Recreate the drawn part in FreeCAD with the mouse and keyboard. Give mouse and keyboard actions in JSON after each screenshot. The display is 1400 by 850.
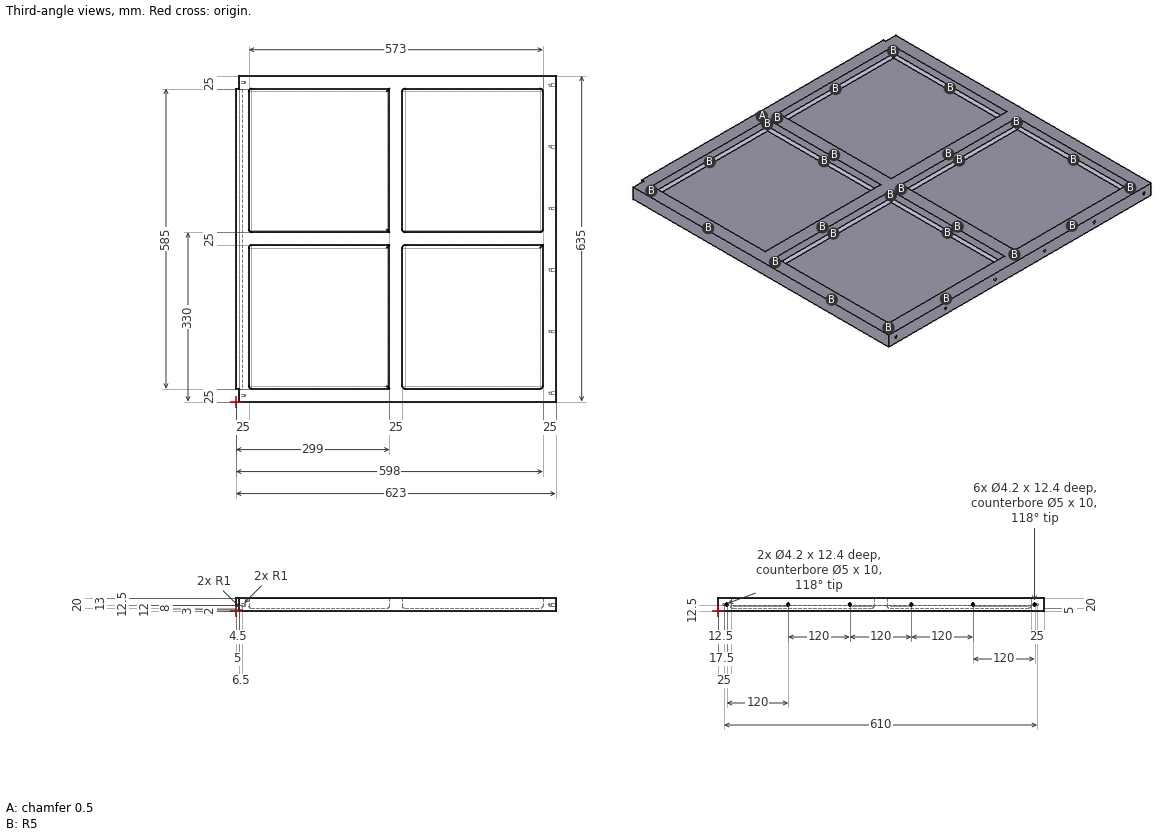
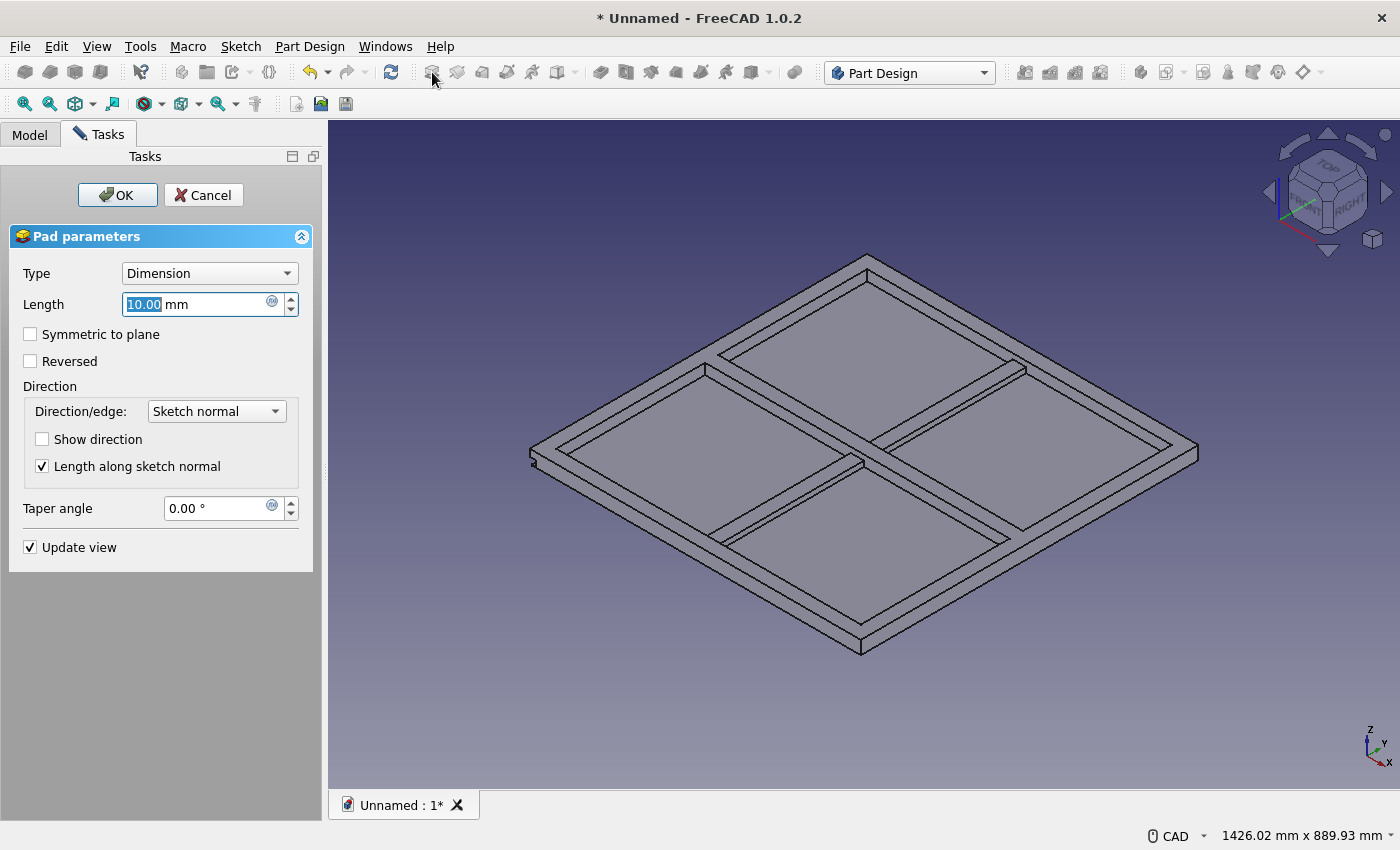
{"action": "type", "text": "20"}
{"action": "key", "text": "Tab"}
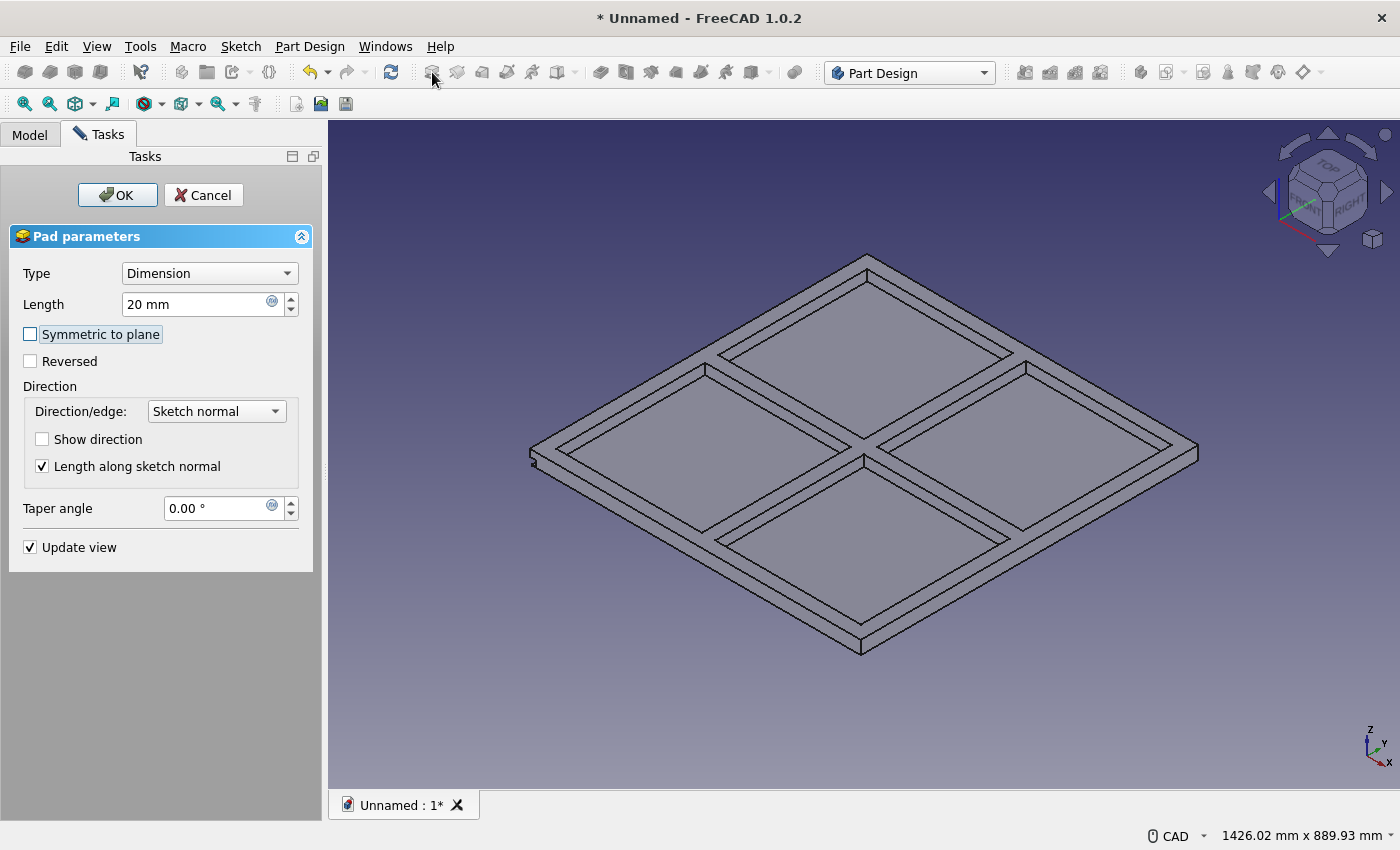
{"action": "left_click", "coordinate": [118, 195]}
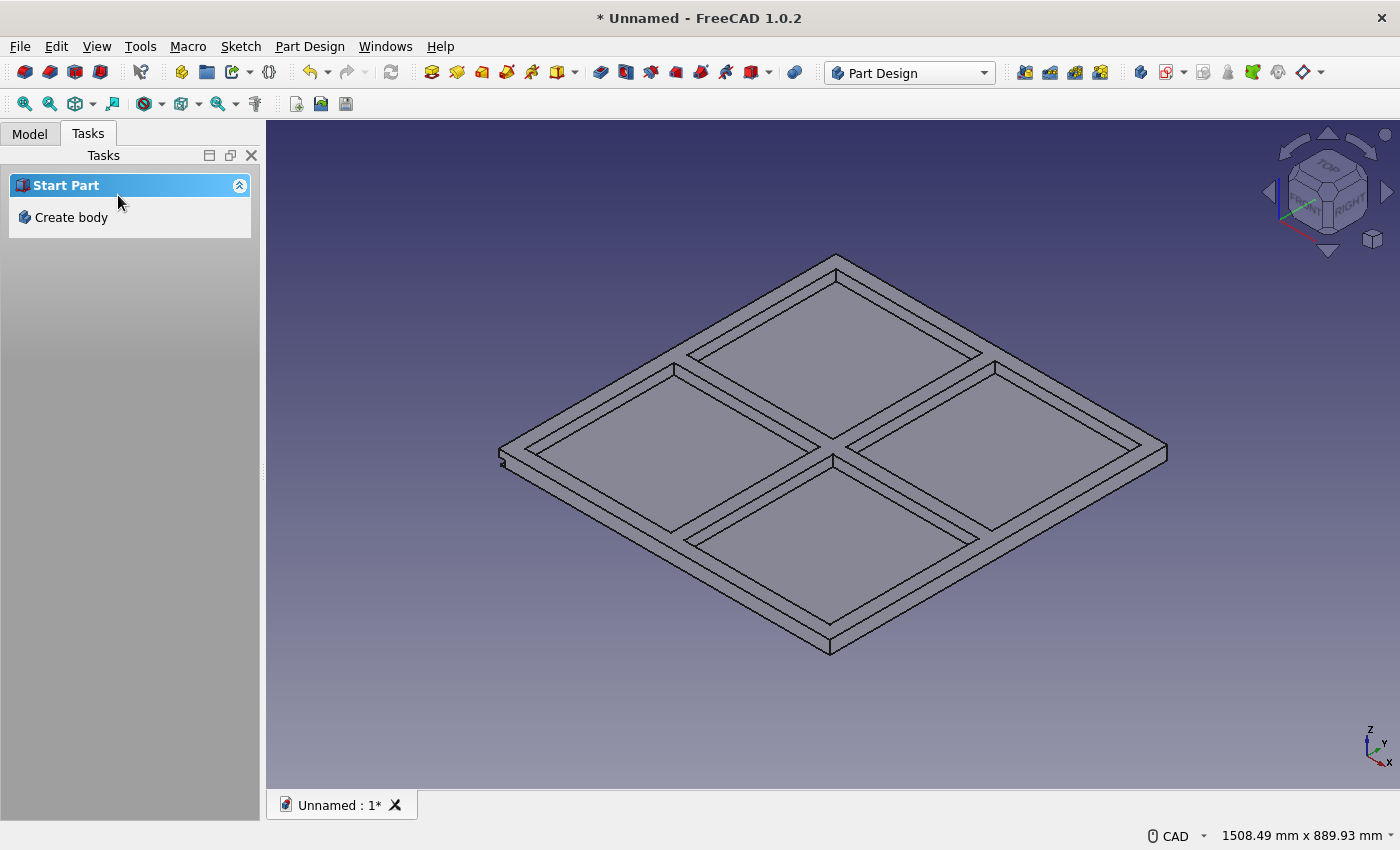
{"action": "key", "text": "4"}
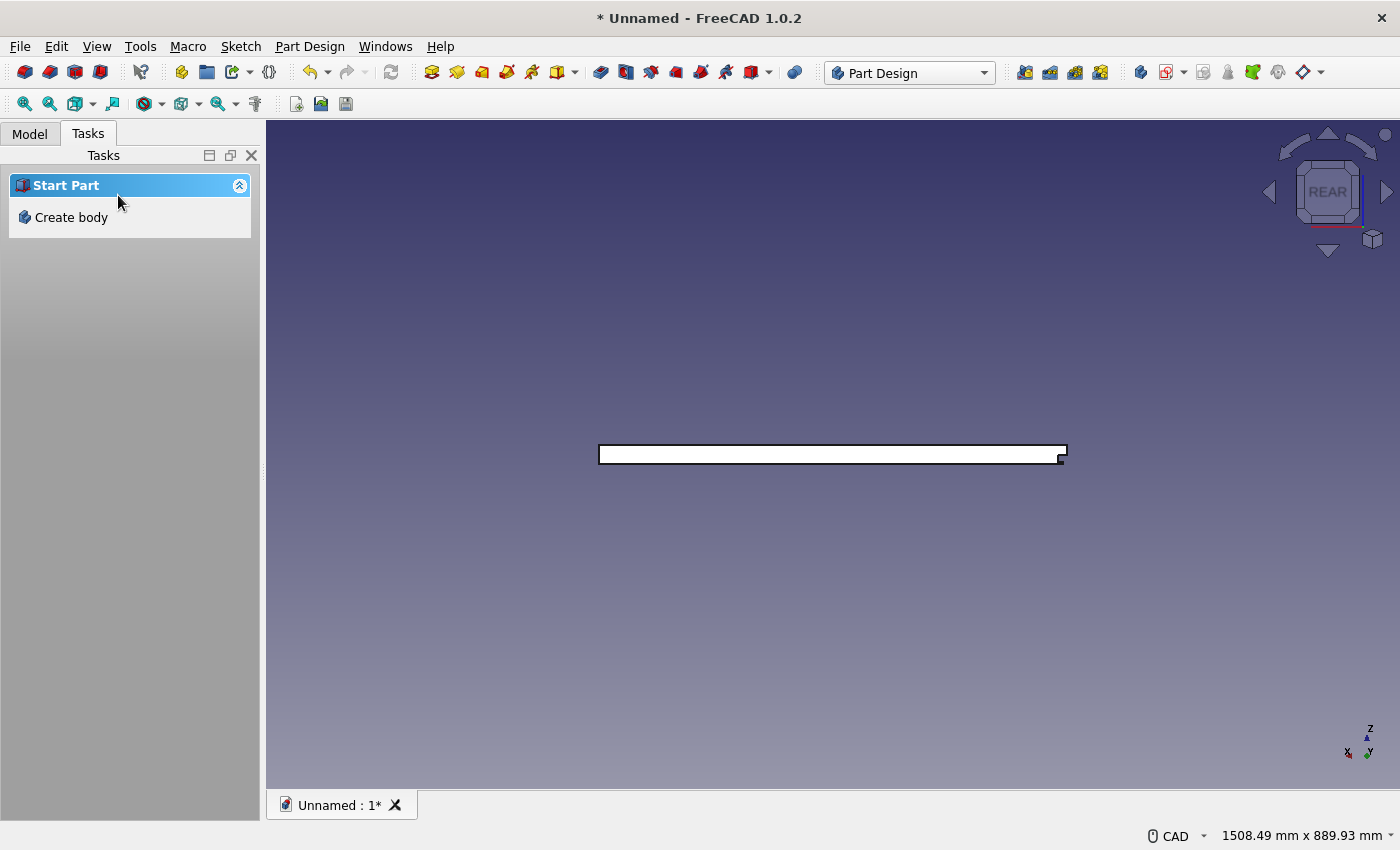
{"action": "left_click", "coordinate": [25, 104]}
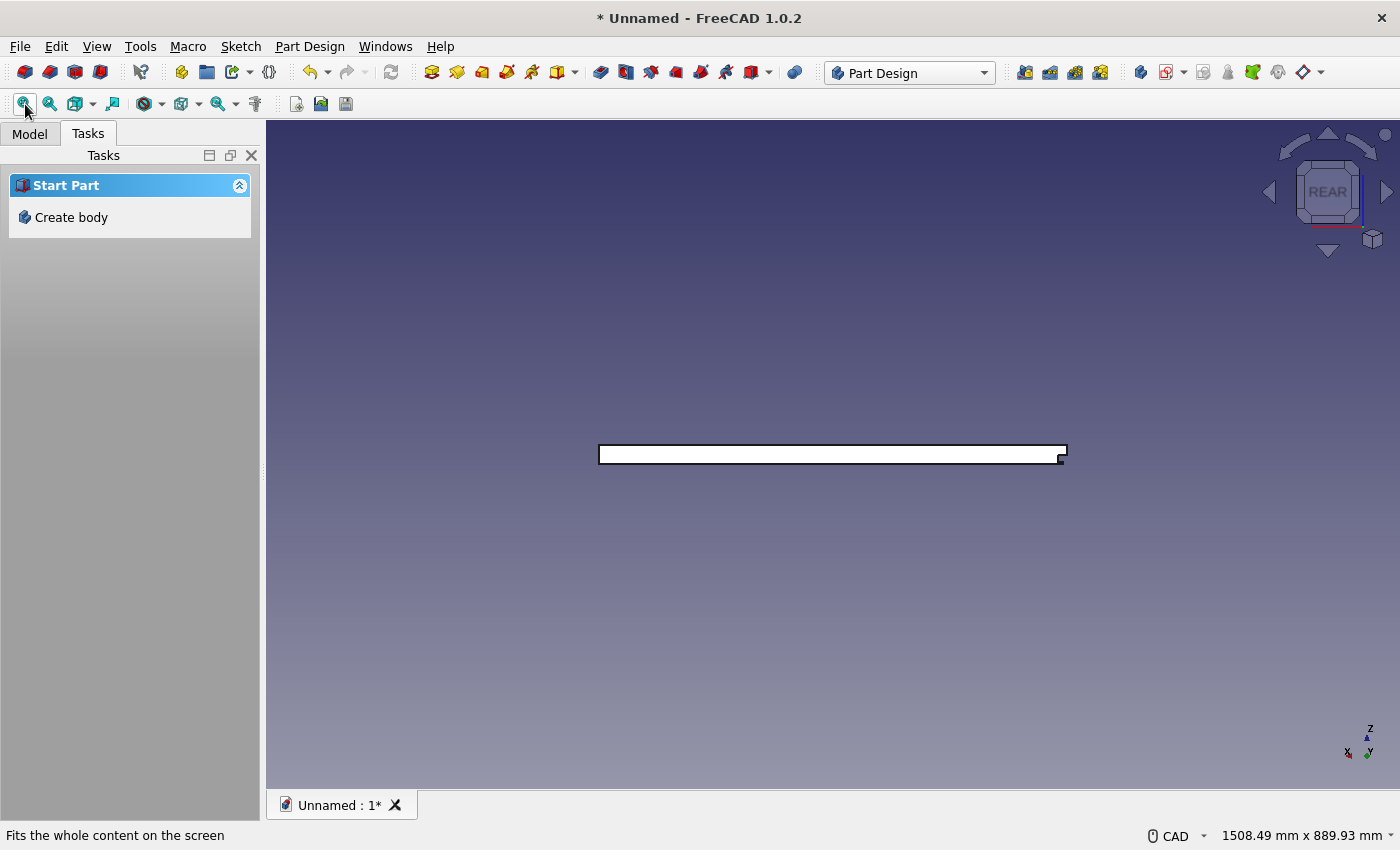
{"action": "left_click", "coordinate": [632, 454]}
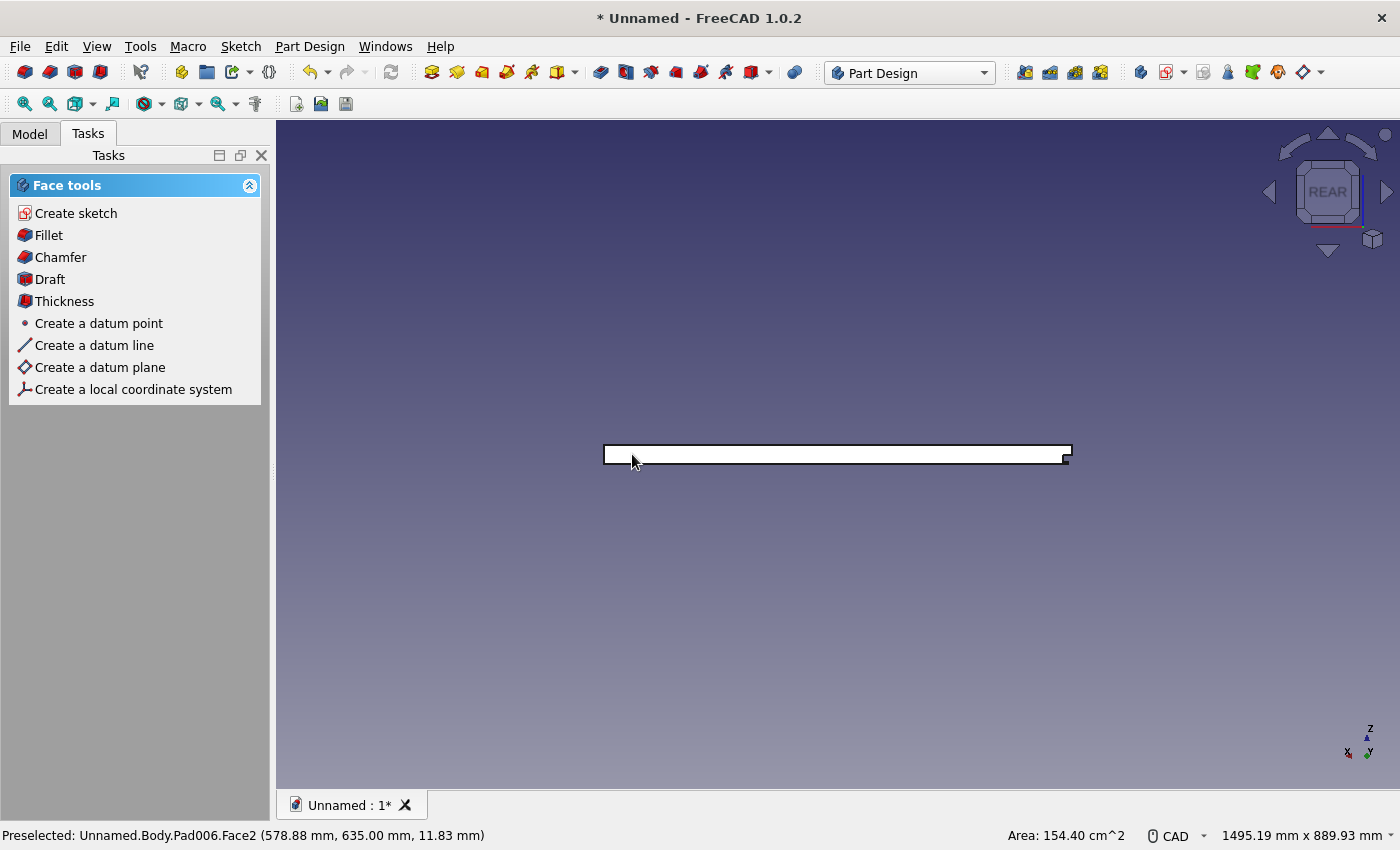
{"action": "left_click", "coordinate": [1166, 72]}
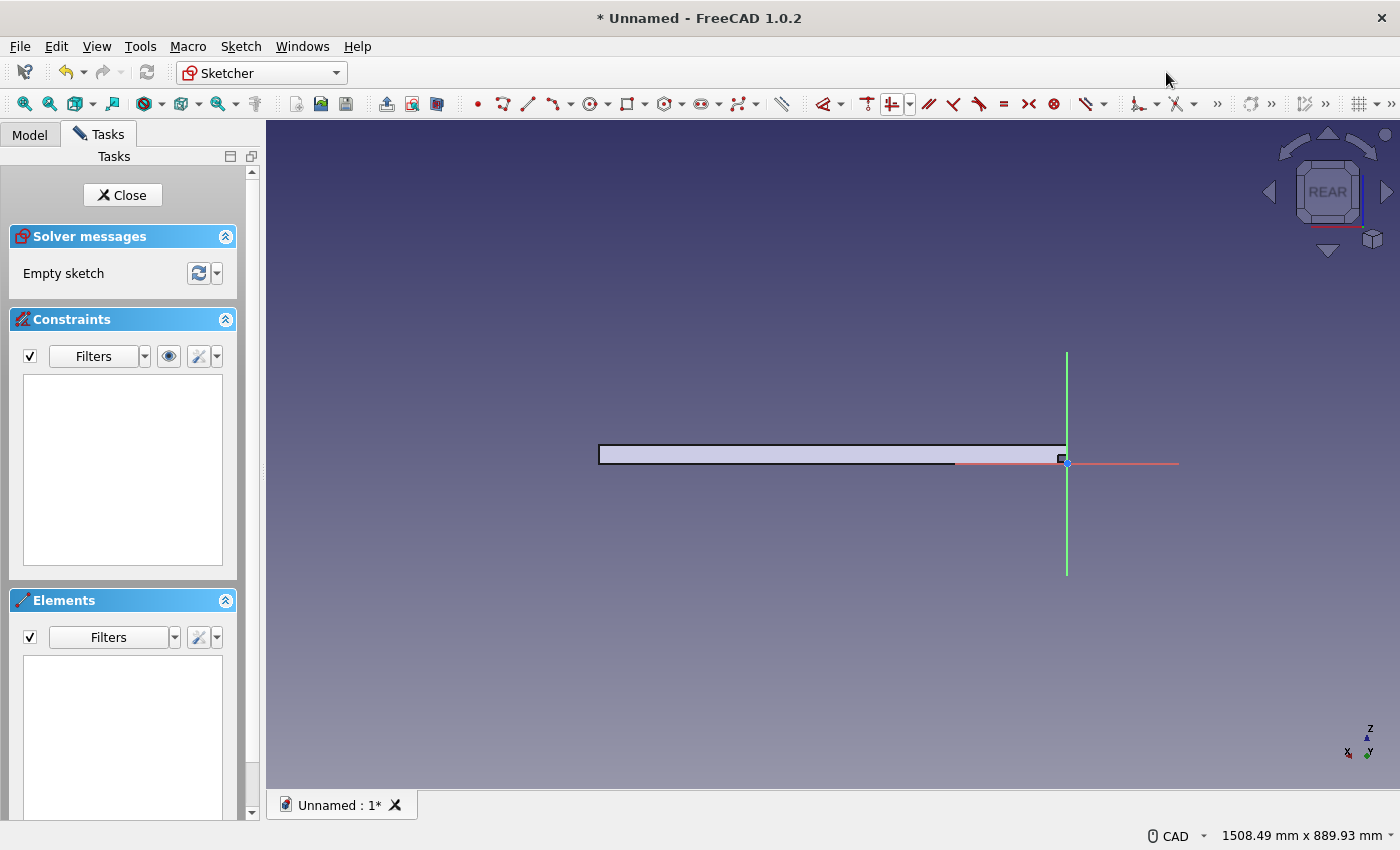
{"action": "scroll", "coordinate": [1078, 460], "scroll_direction": "up", "scroll_amount": 15}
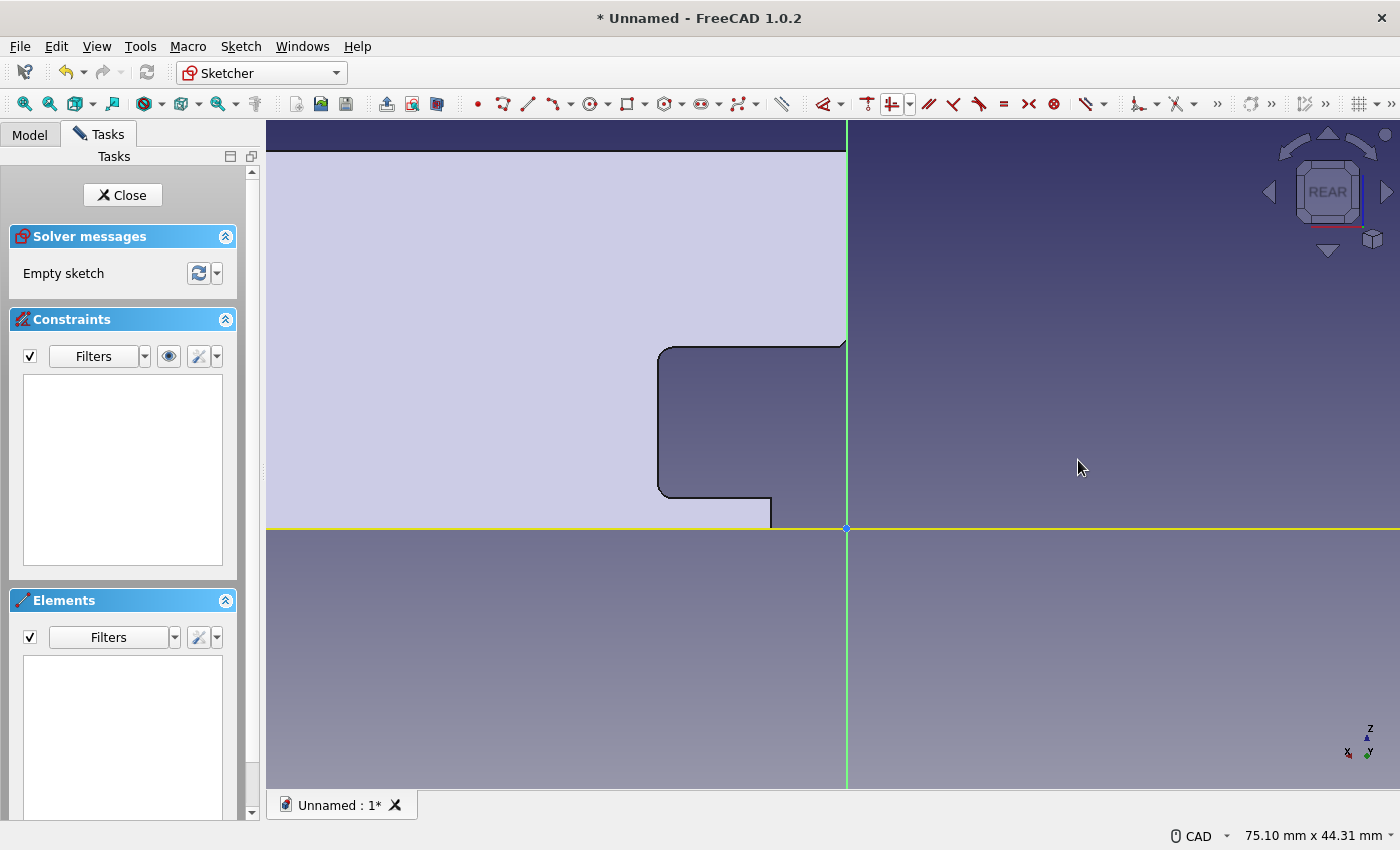
{"action": "scroll", "coordinate": [742, 424], "scroll_direction": "up", "scroll_amount": 4}